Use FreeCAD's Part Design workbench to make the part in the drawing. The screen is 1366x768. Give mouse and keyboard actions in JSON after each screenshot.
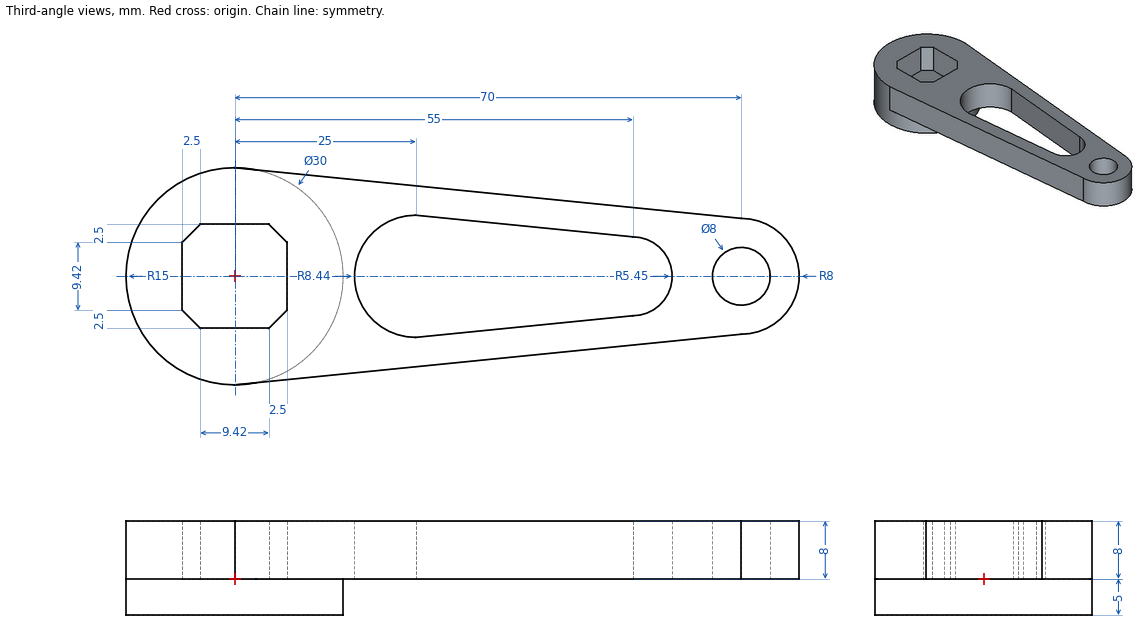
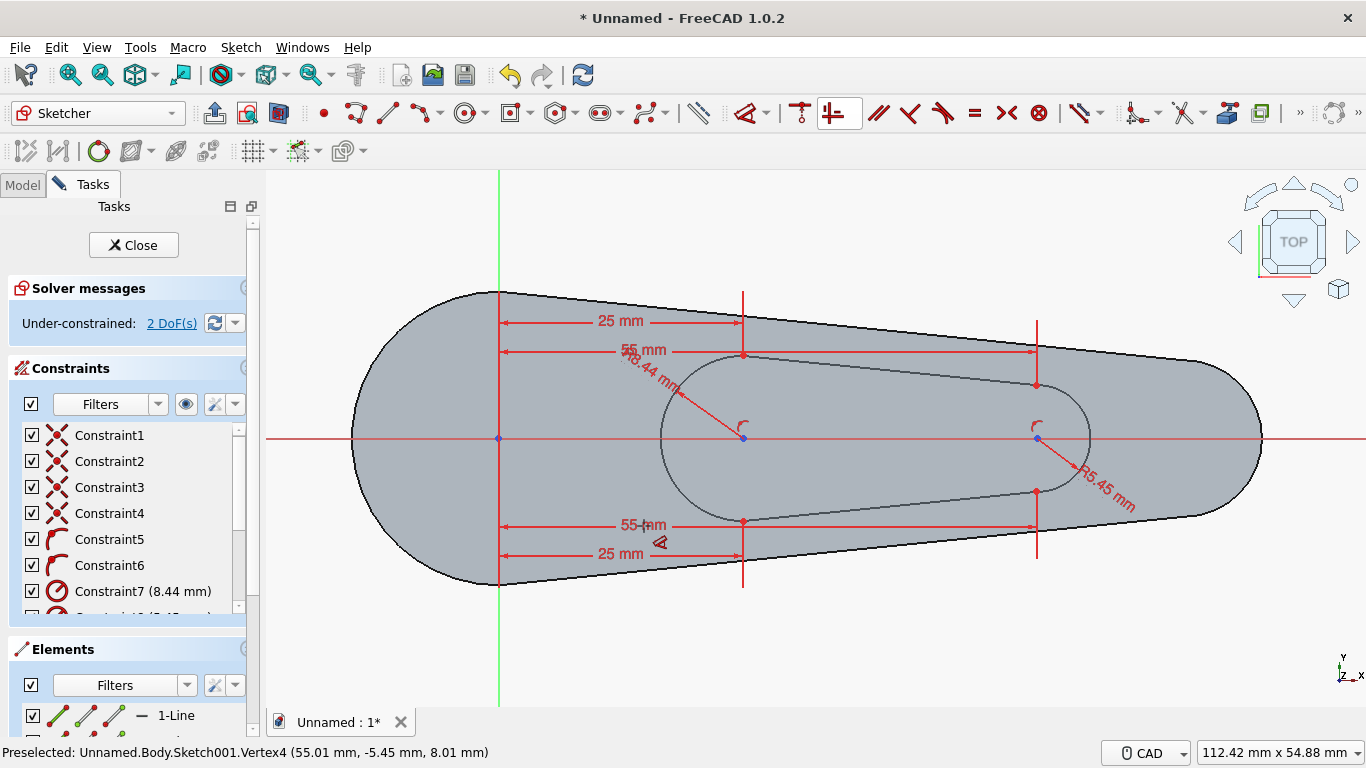
{"action": "left_click", "coordinate": [743, 438]}
{"action": "left_click", "coordinate": [621, 472]}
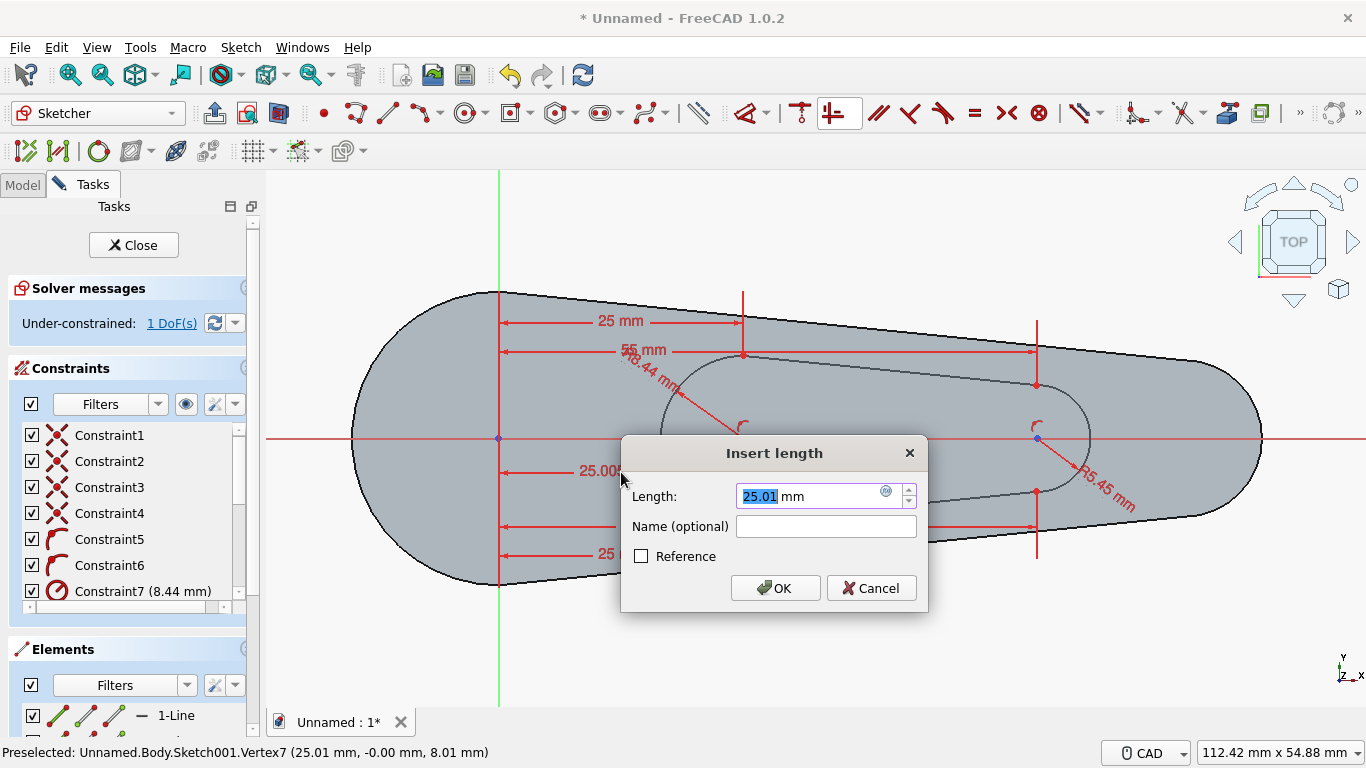
{"action": "type", "text": "25"}
{"action": "key", "text": "Return"}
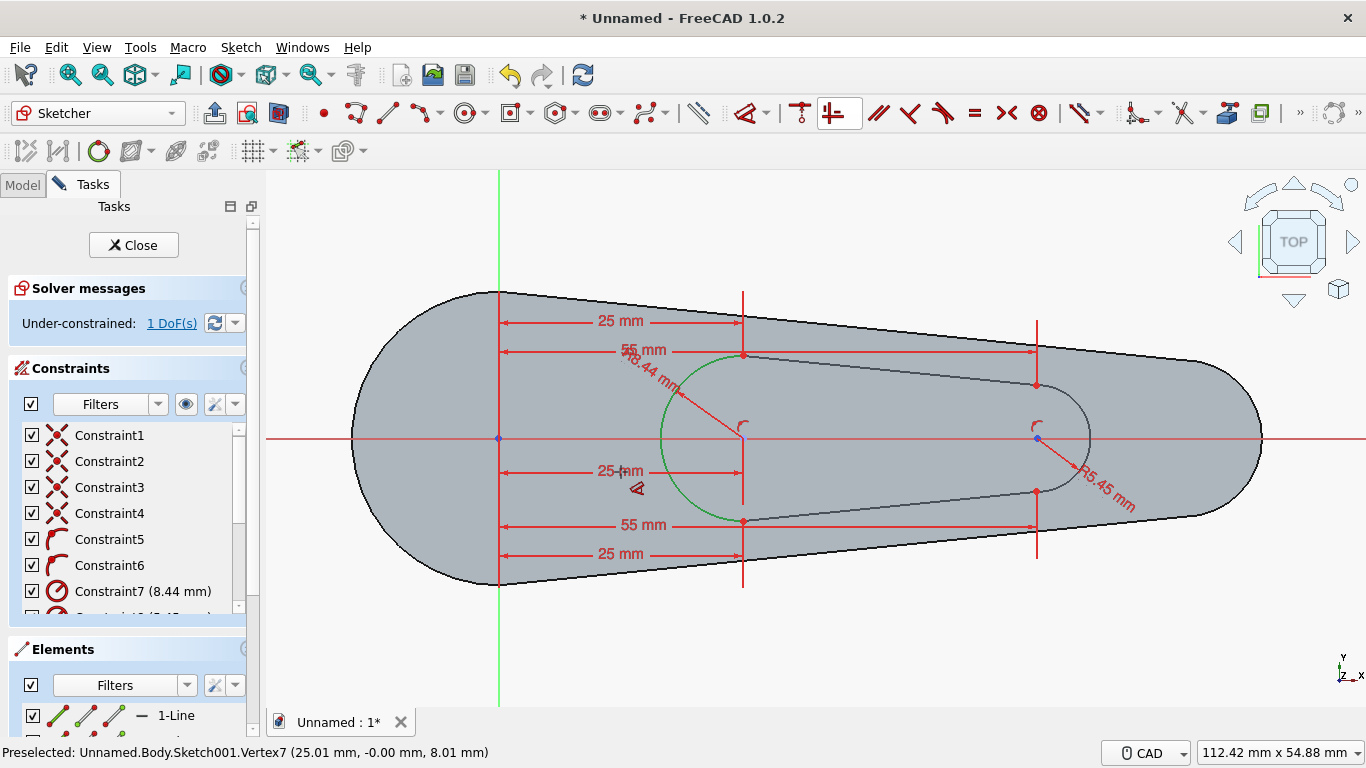
{"action": "left_click", "coordinate": [1037, 438]}
{"action": "left_click", "coordinate": [768, 472]}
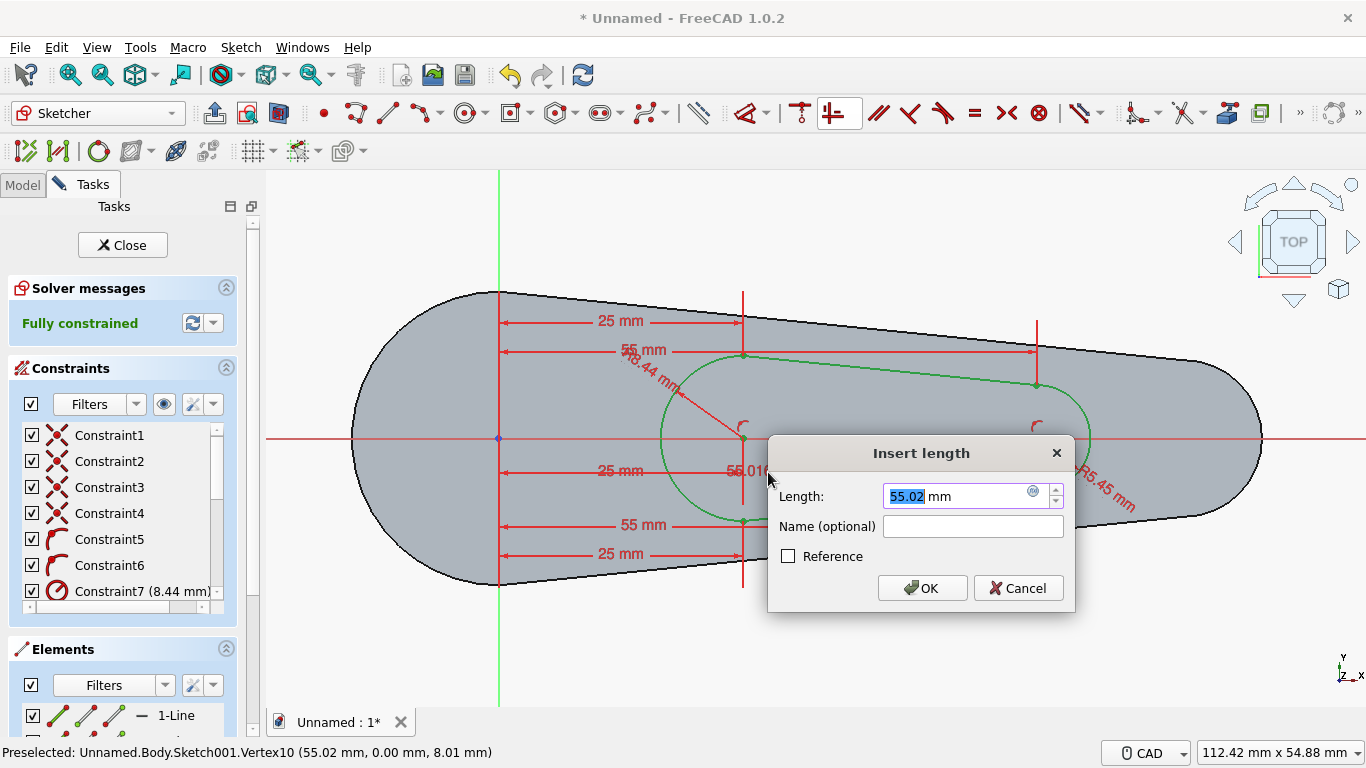
{"action": "type", "text": "55"}
{"action": "key", "text": "Return"}
{"action": "key", "text": "Escape"}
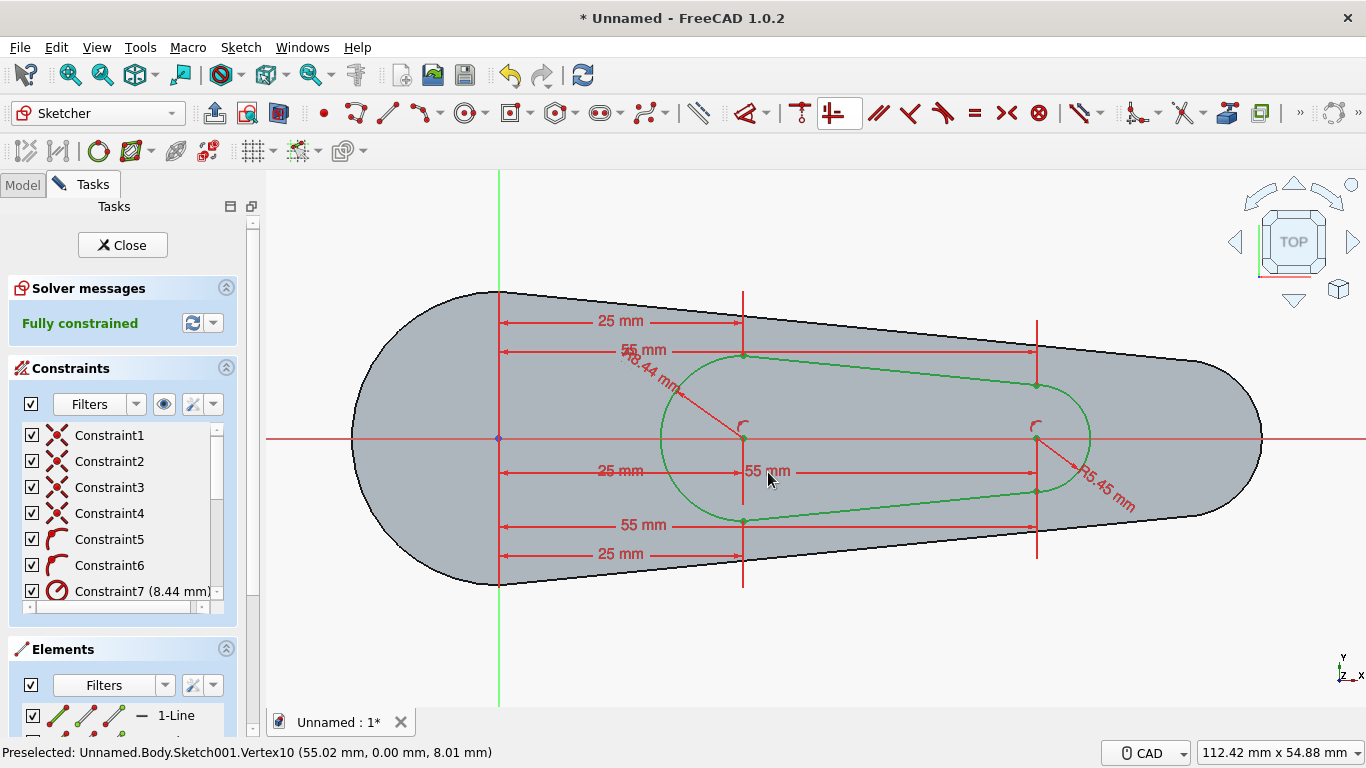
{"action": "left_click", "coordinate": [123, 245]}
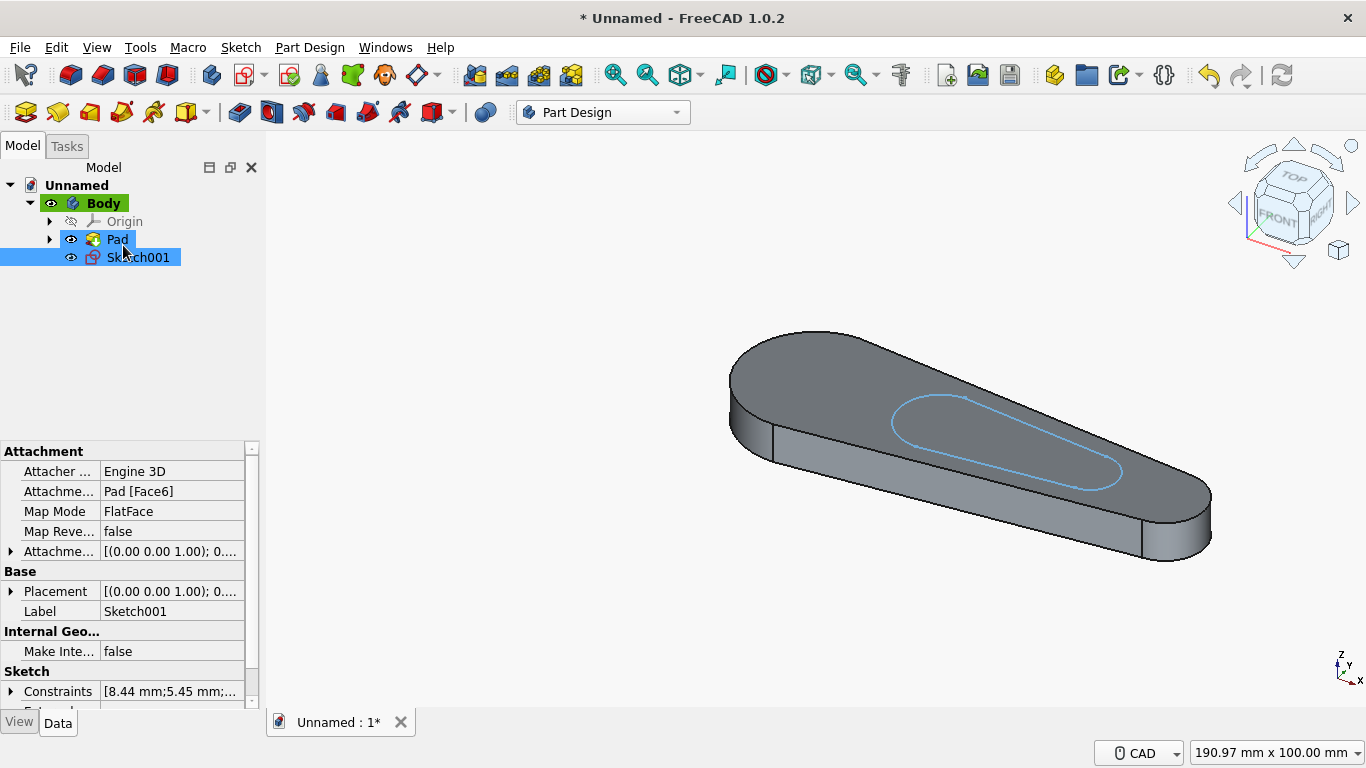
{"action": "left_click", "coordinate": [240, 112]}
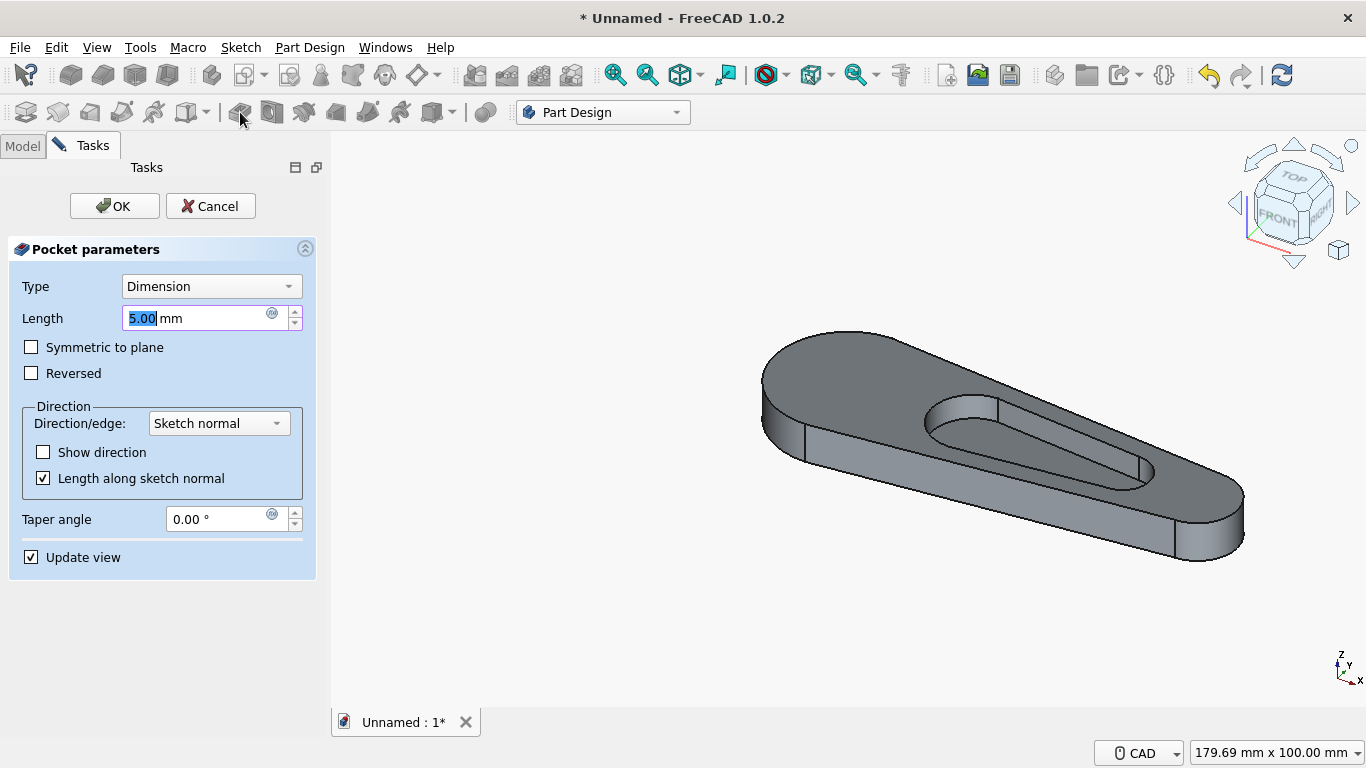
{"action": "type", "text": "8"}
{"action": "key", "text": "Tab"}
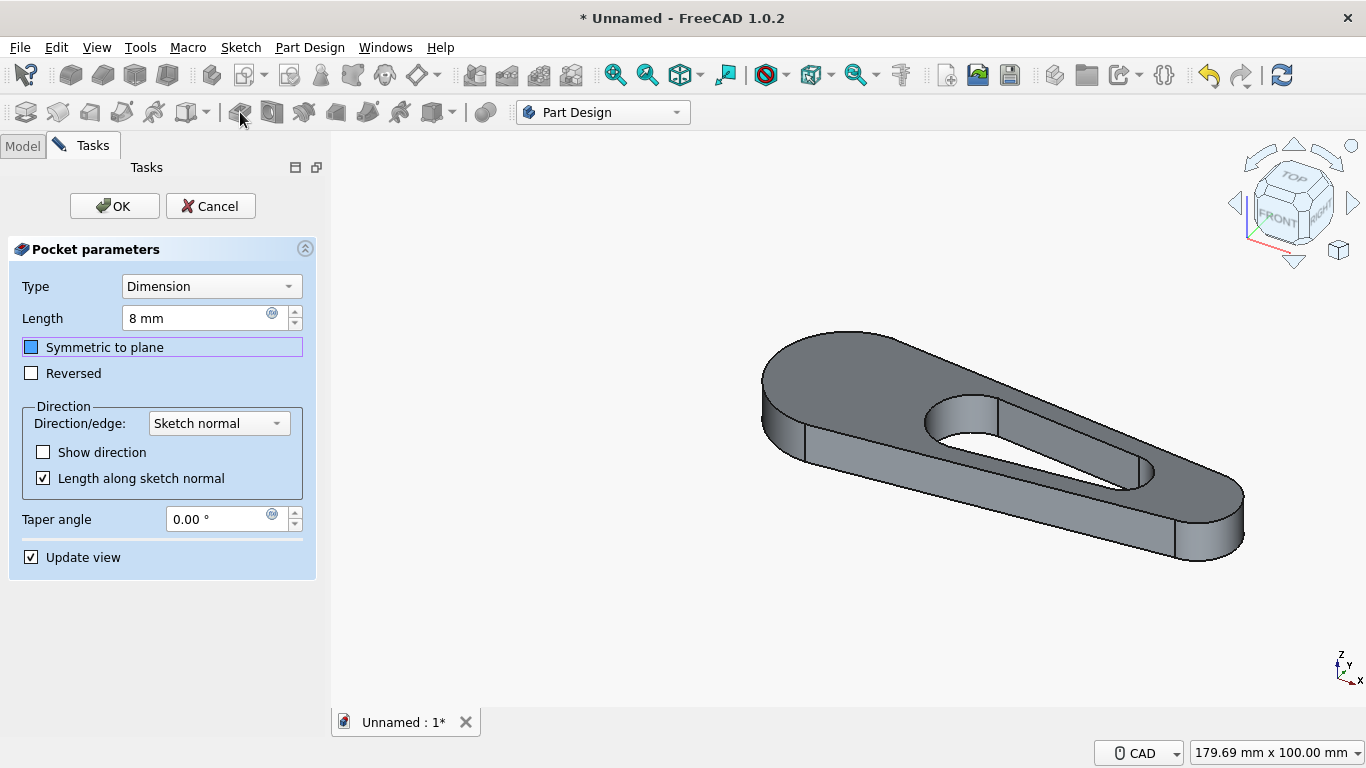
{"action": "left_click", "coordinate": [115, 206]}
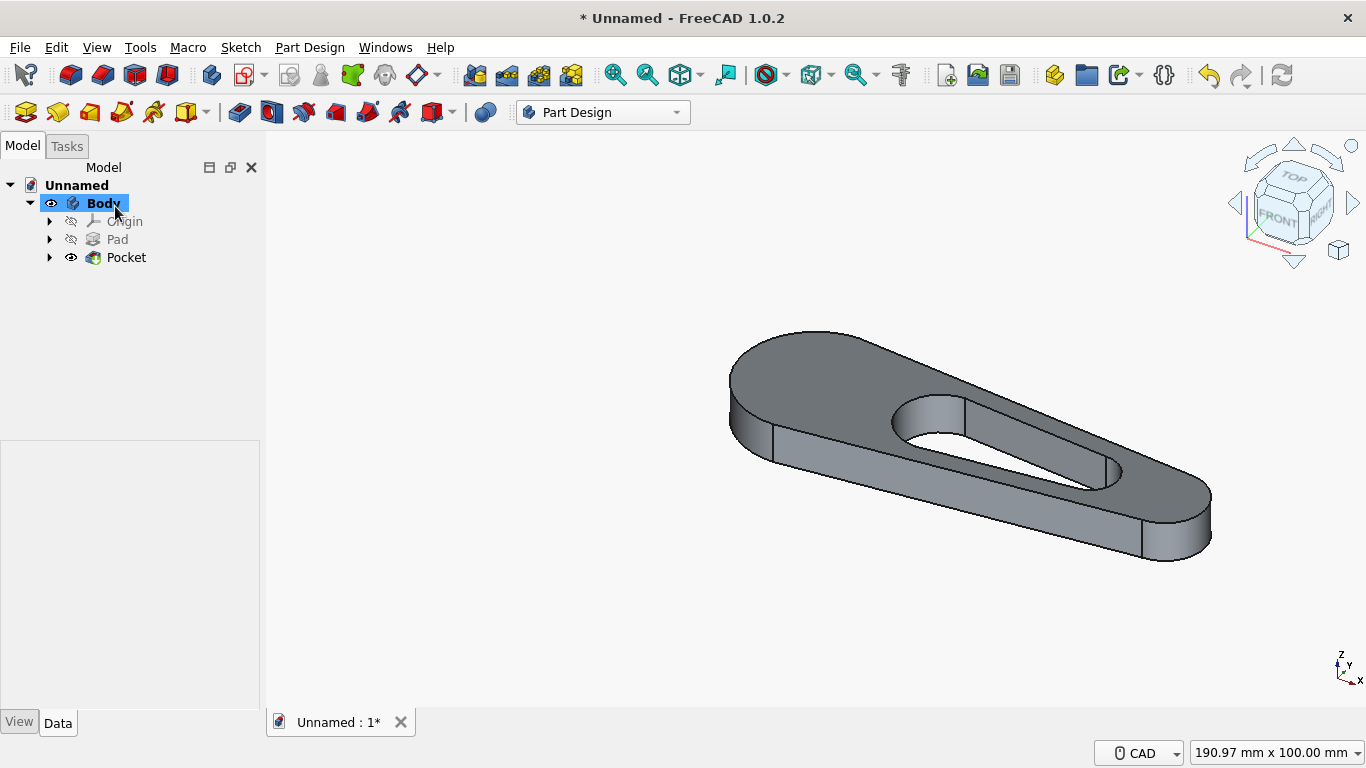
{"action": "left_click", "coordinate": [50, 221]}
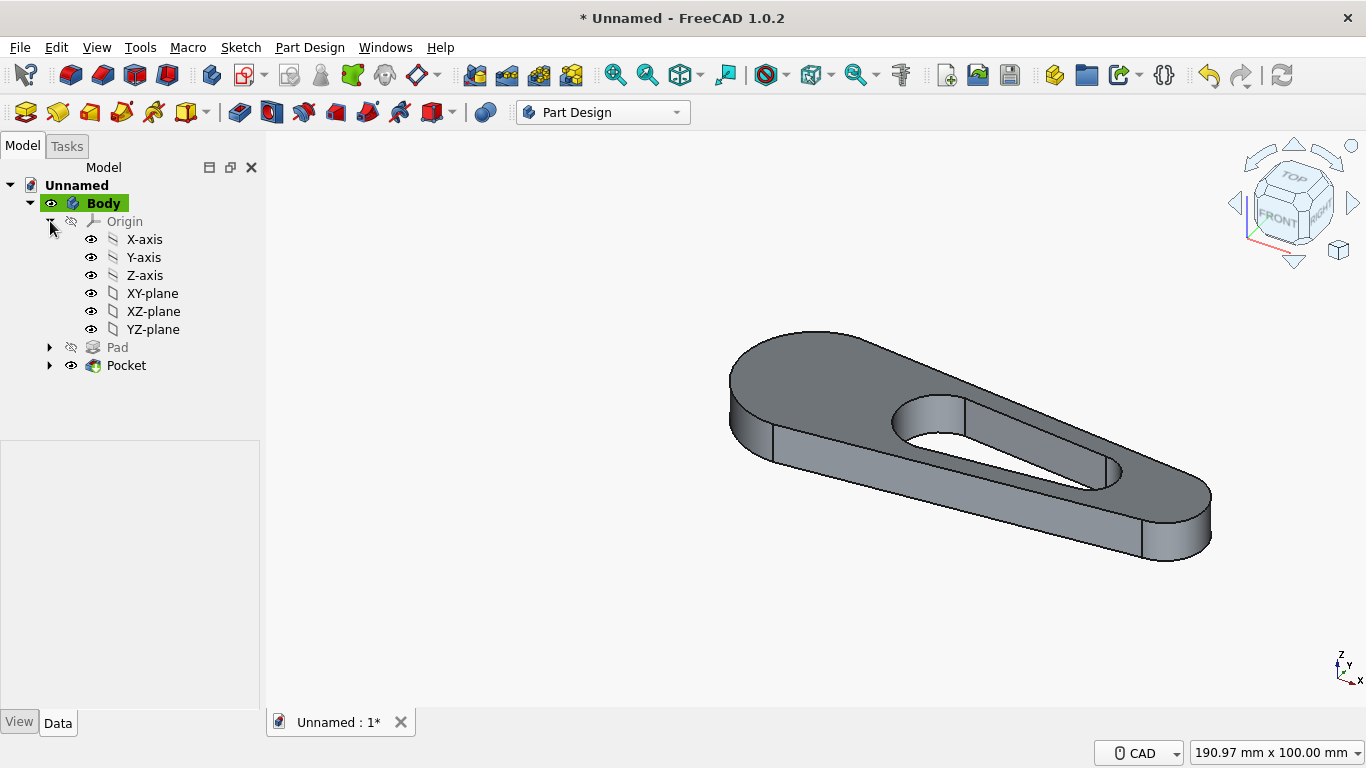
{"action": "left_click", "coordinate": [136, 293]}